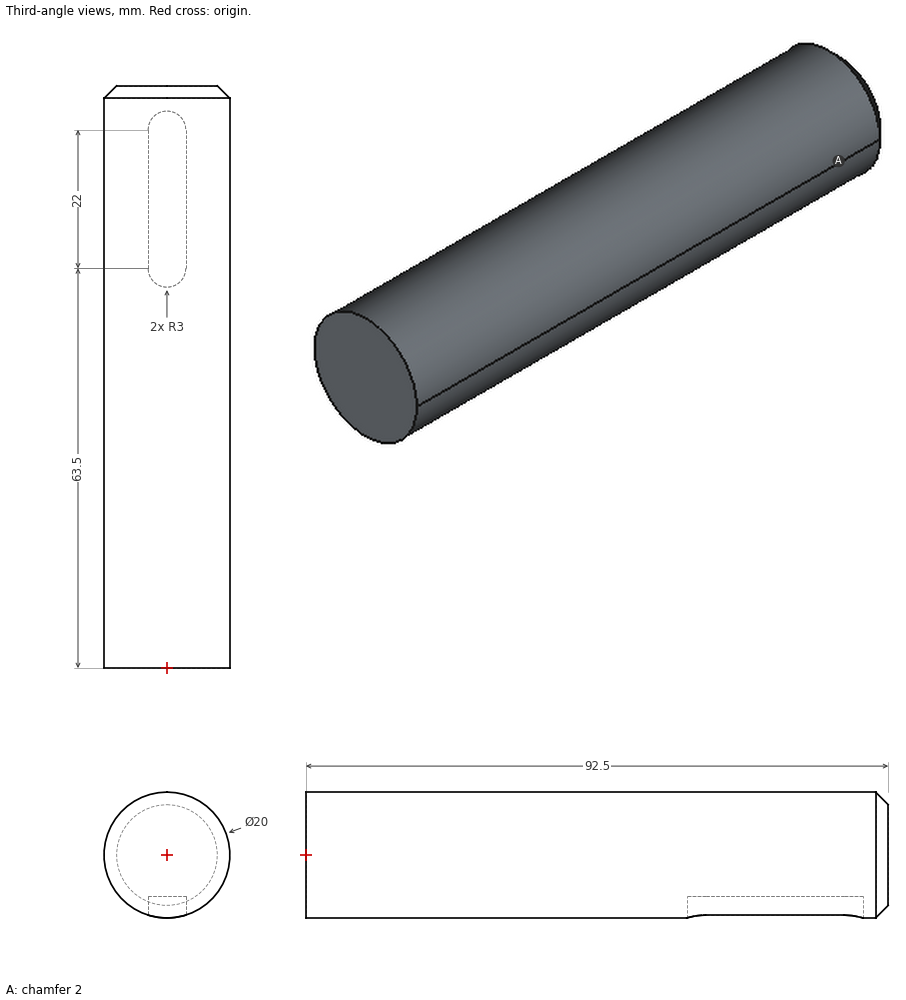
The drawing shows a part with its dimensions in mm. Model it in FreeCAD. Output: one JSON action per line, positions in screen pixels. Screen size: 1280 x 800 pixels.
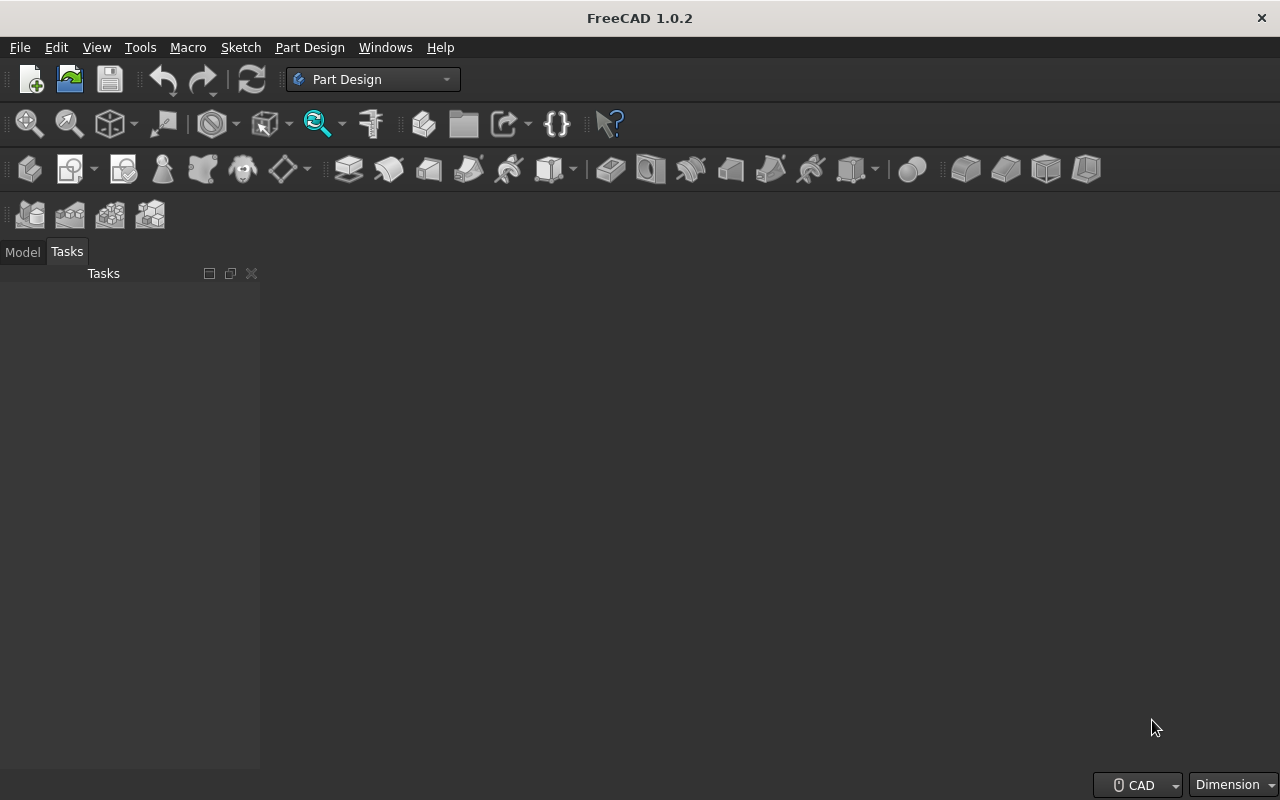
{"action": "left_click", "coordinate": [30, 80]}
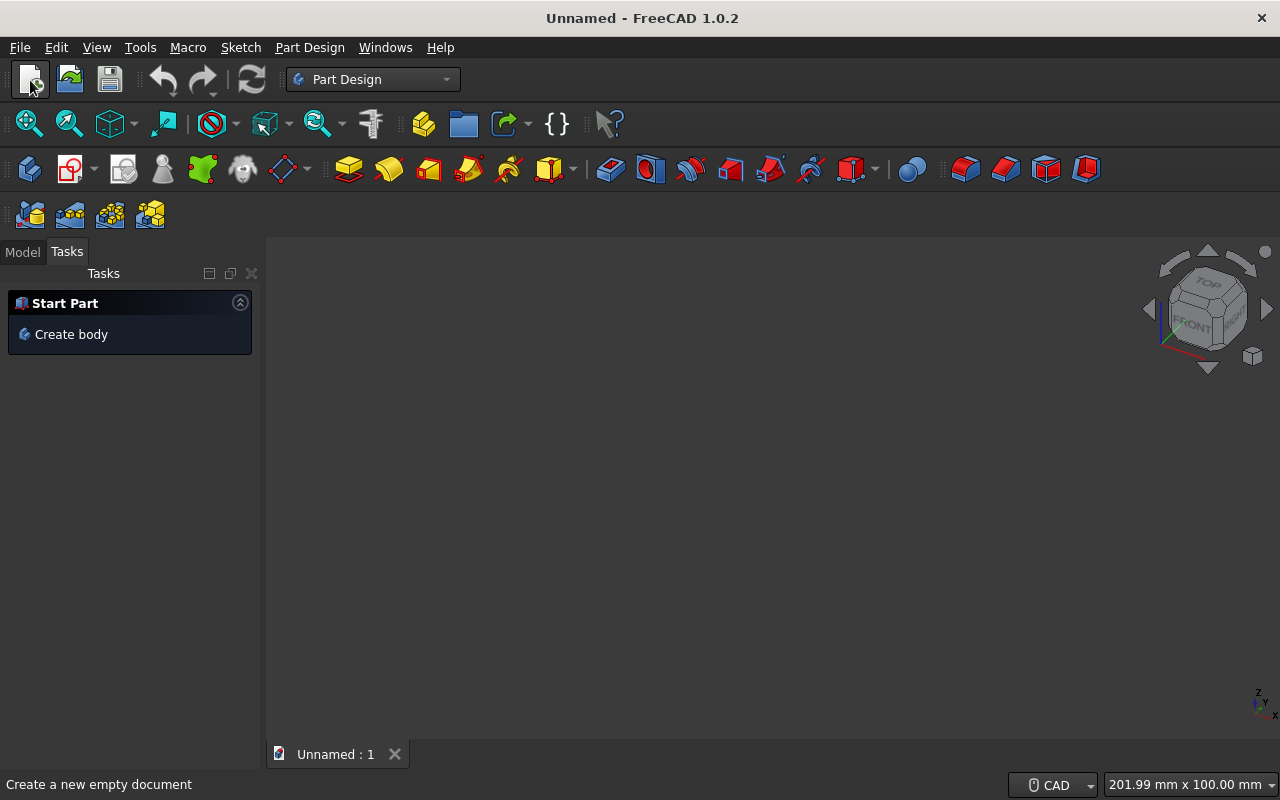
{"action": "left_click", "coordinate": [70, 170]}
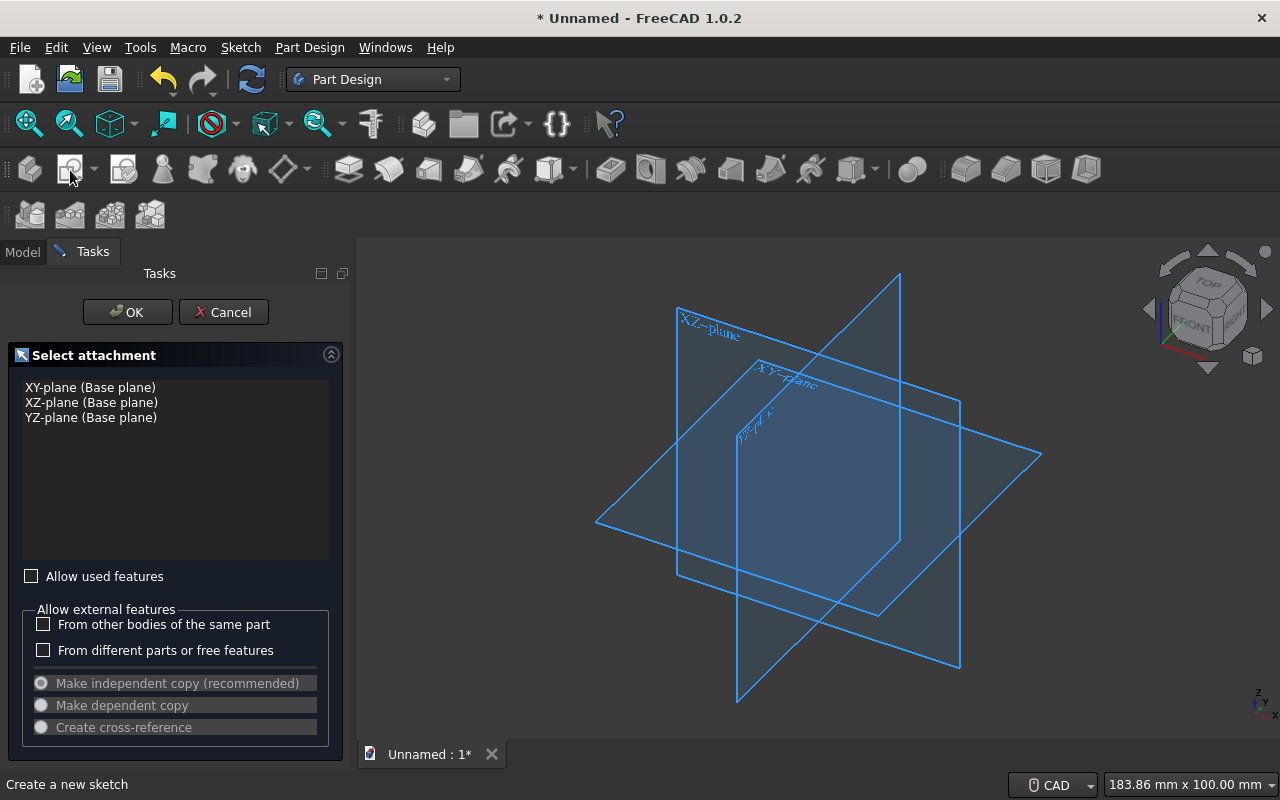
{"action": "left_click", "coordinate": [82, 402]}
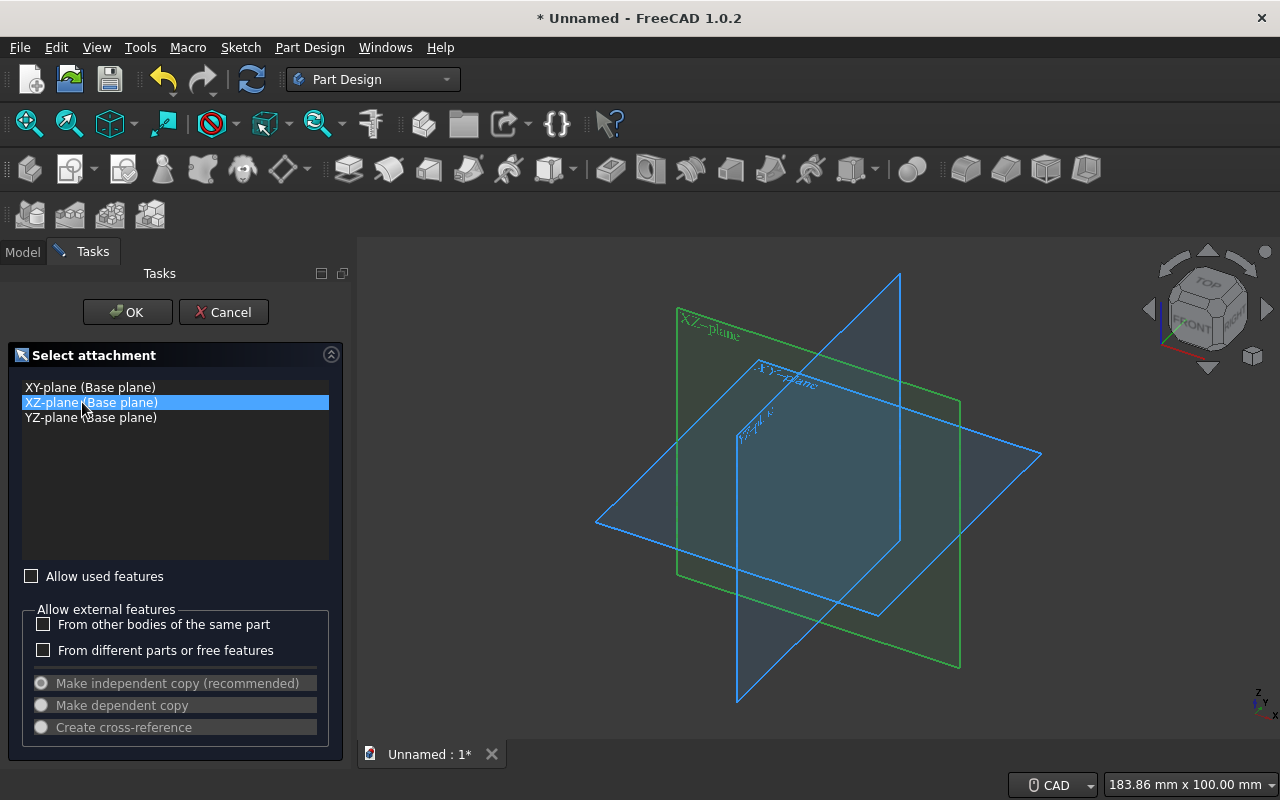
{"action": "left_click", "coordinate": [128, 312]}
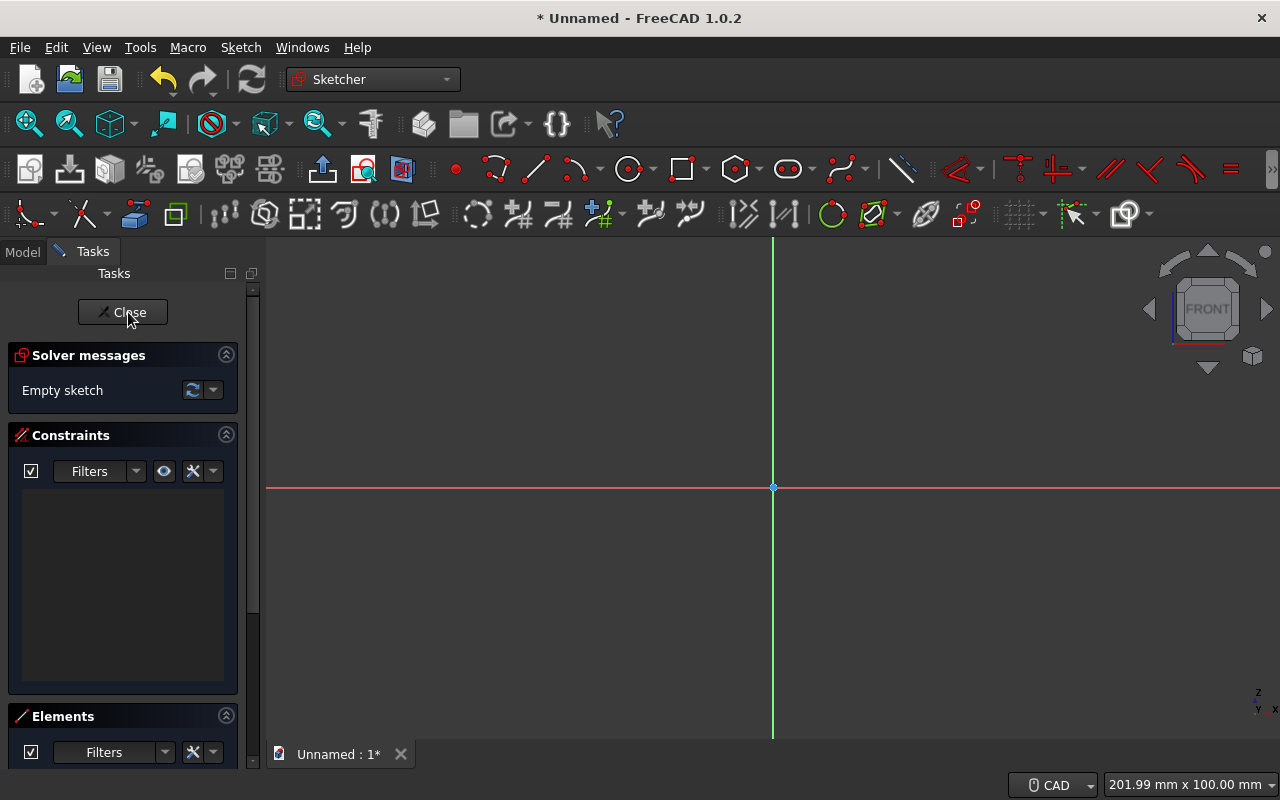
{"action": "scroll", "coordinate": [803, 488], "scroll_direction": "up", "scroll_amount": 6}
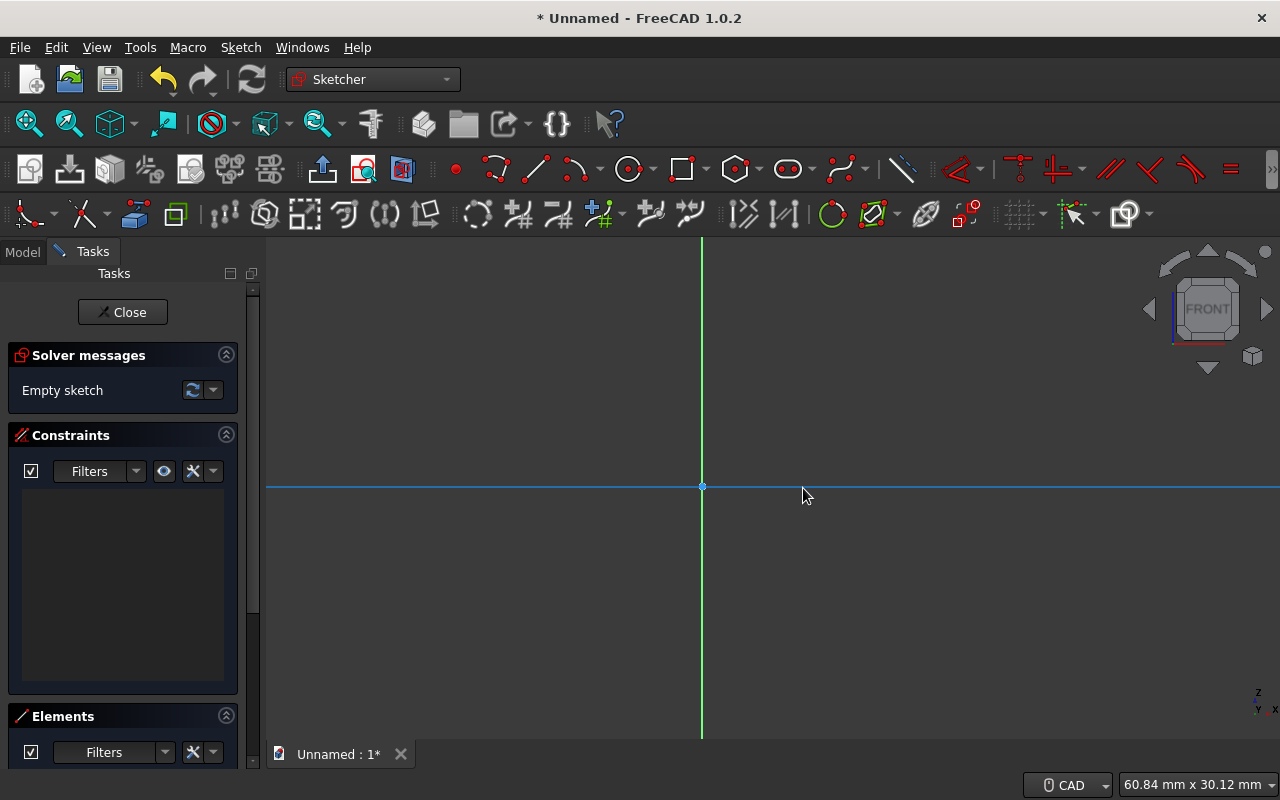
{"action": "left_click", "coordinate": [630, 170]}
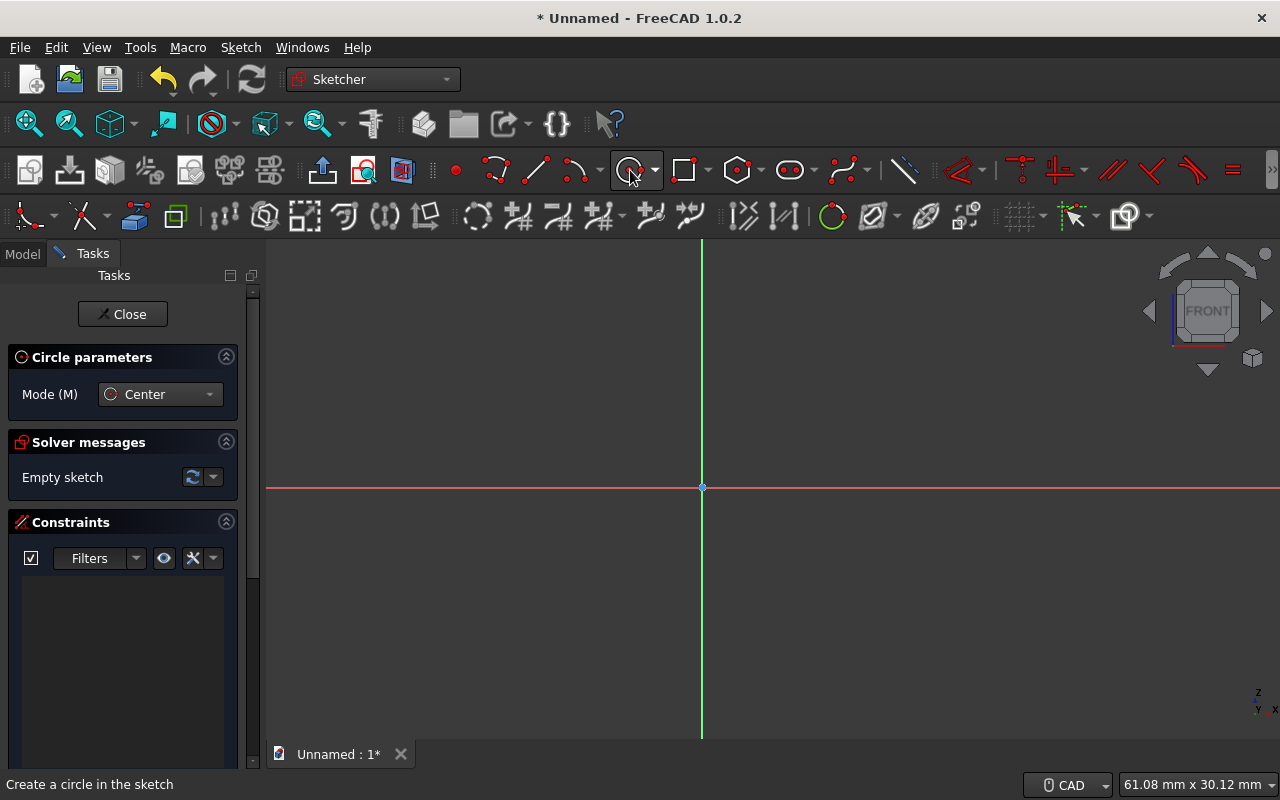
{"action": "left_click", "coordinate": [702, 488]}
{"action": "left_click", "coordinate": [820, 370]}
{"action": "key", "text": "Escape"}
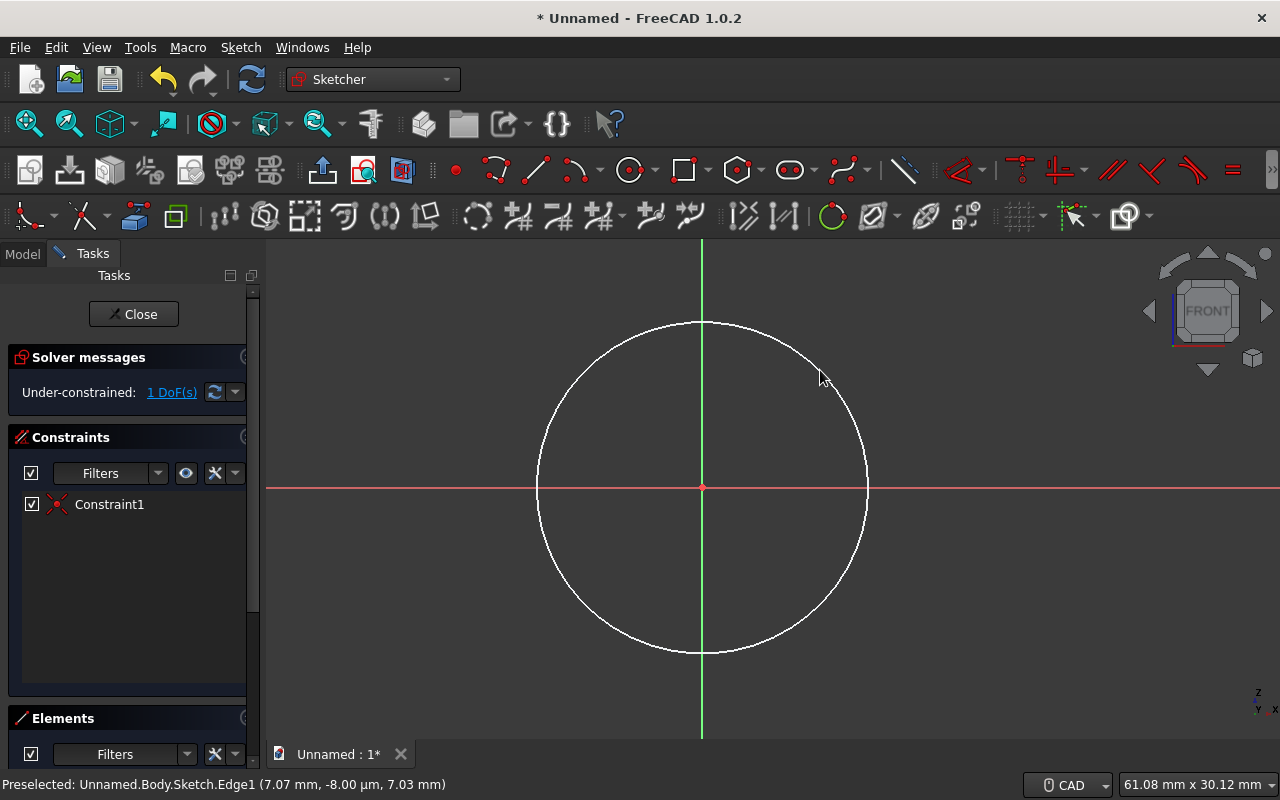
{"action": "key", "text": "d"}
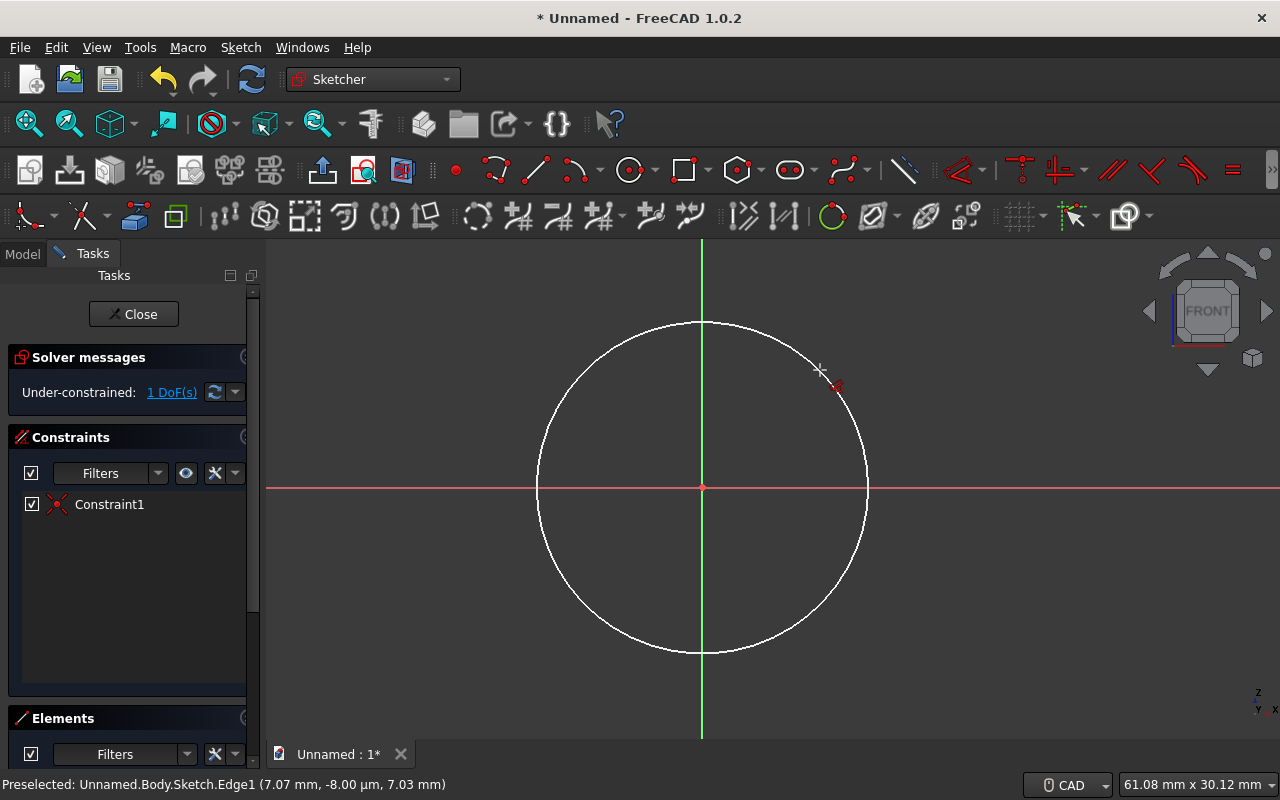
{"action": "left_click", "coordinate": [819, 370]}
{"action": "left_click", "coordinate": [842, 347]}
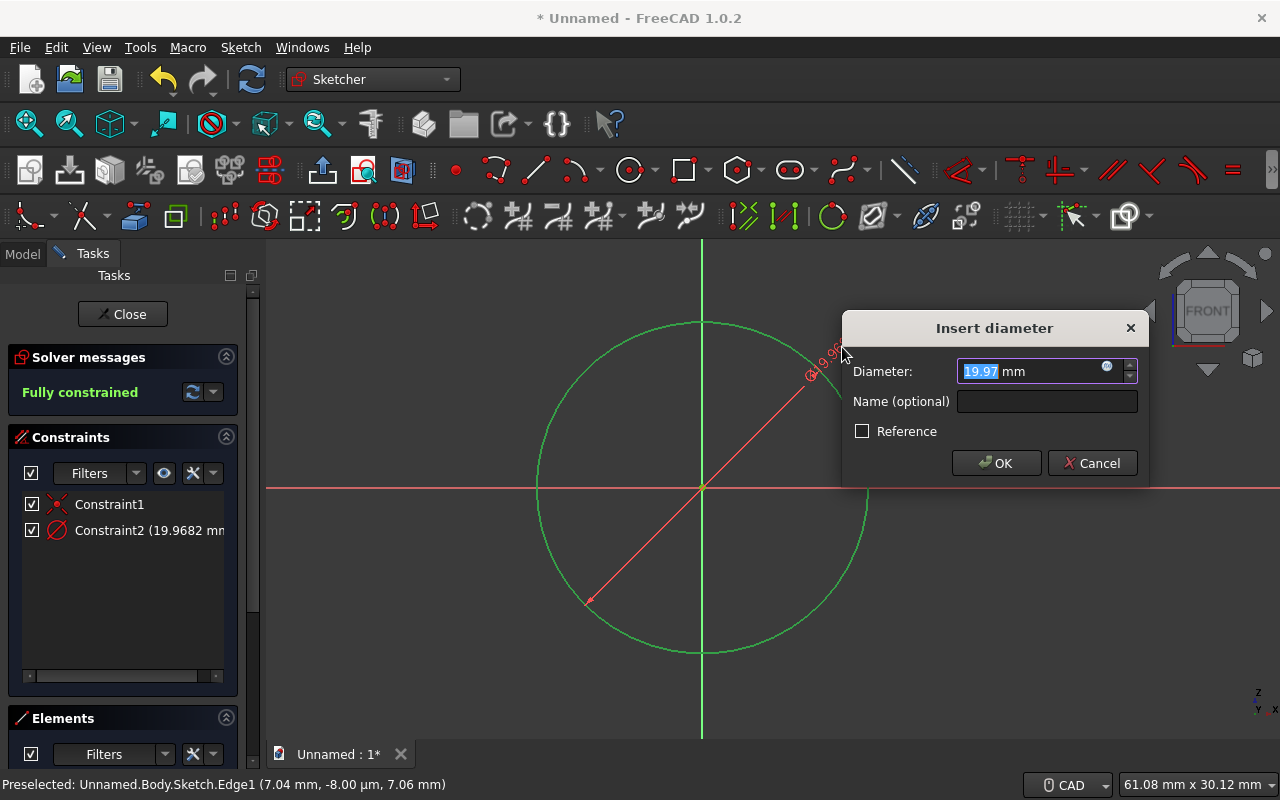
{"action": "type", "text": "20"}
{"action": "key", "text": "Return"}
{"action": "key", "text": "Escape"}